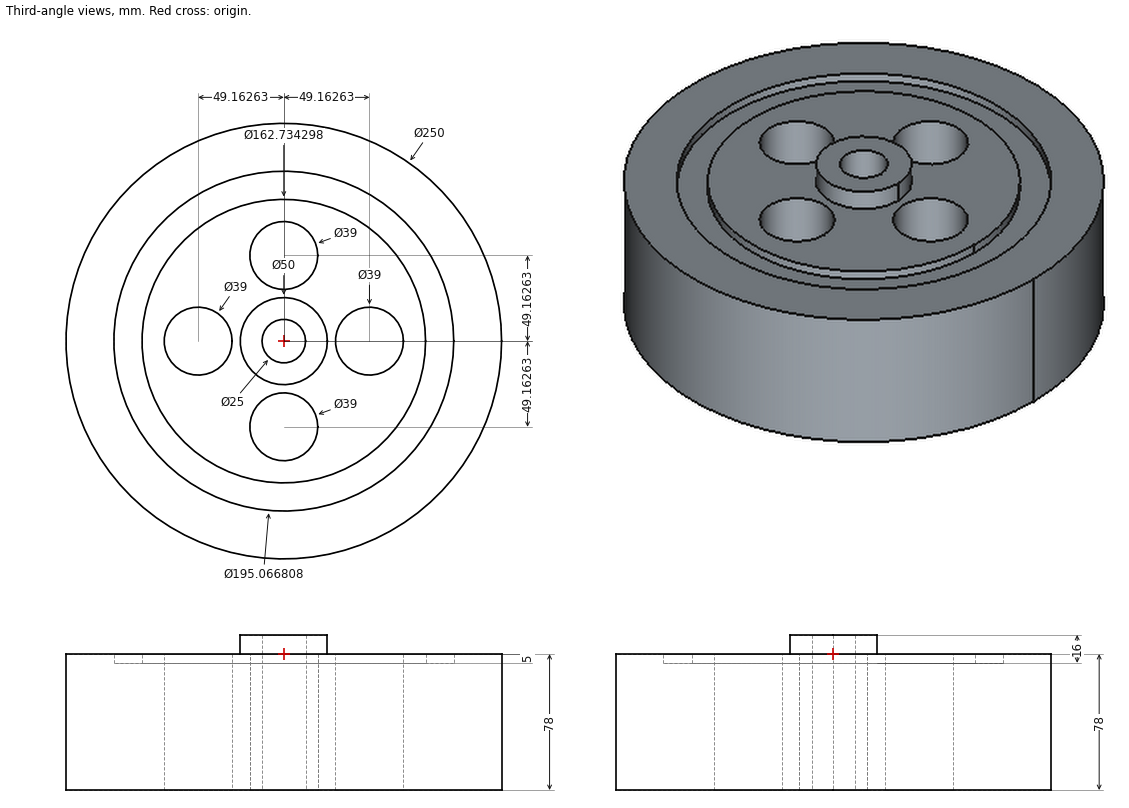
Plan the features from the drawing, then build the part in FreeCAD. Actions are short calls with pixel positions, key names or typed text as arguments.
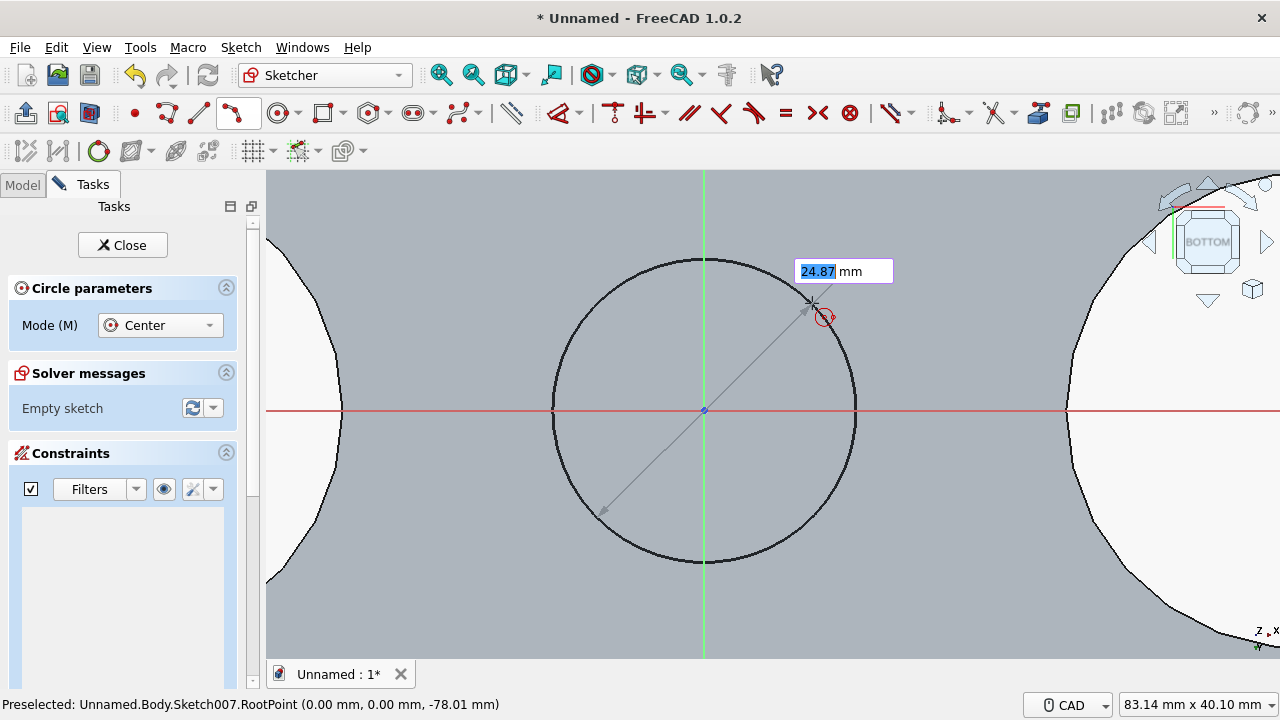
text(25)
key(Return)
key(Escape)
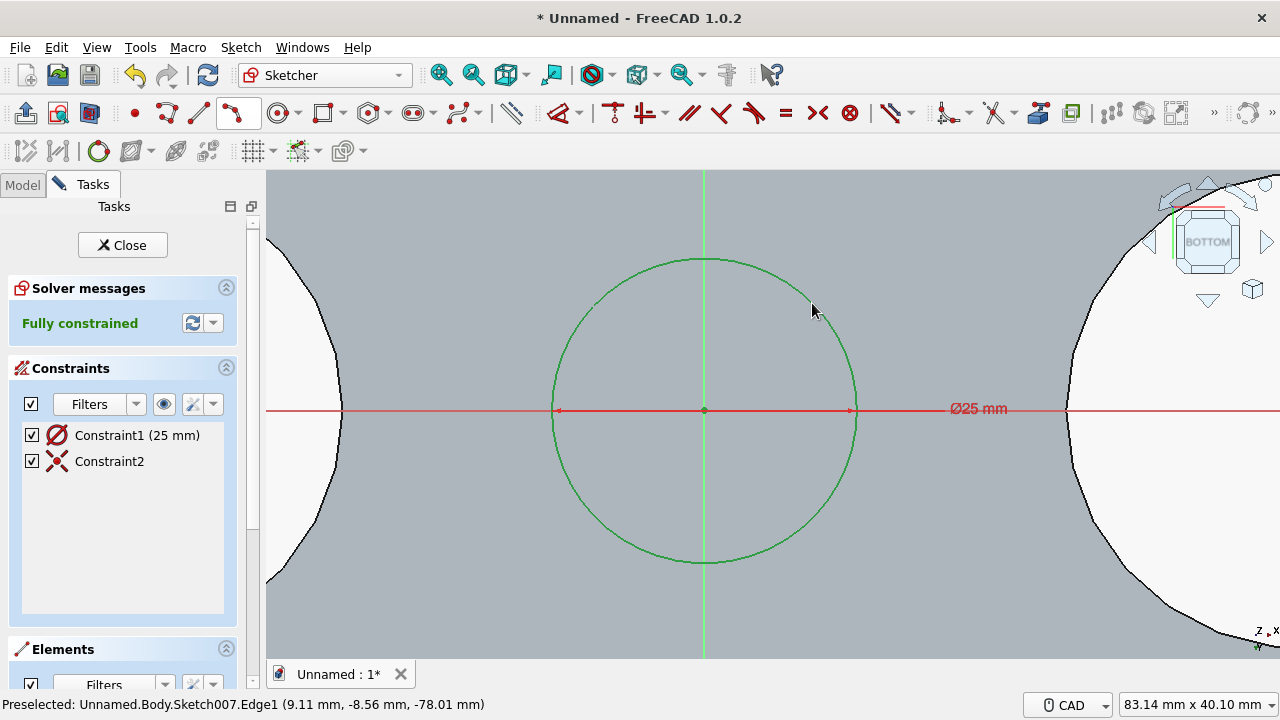
click(123, 245)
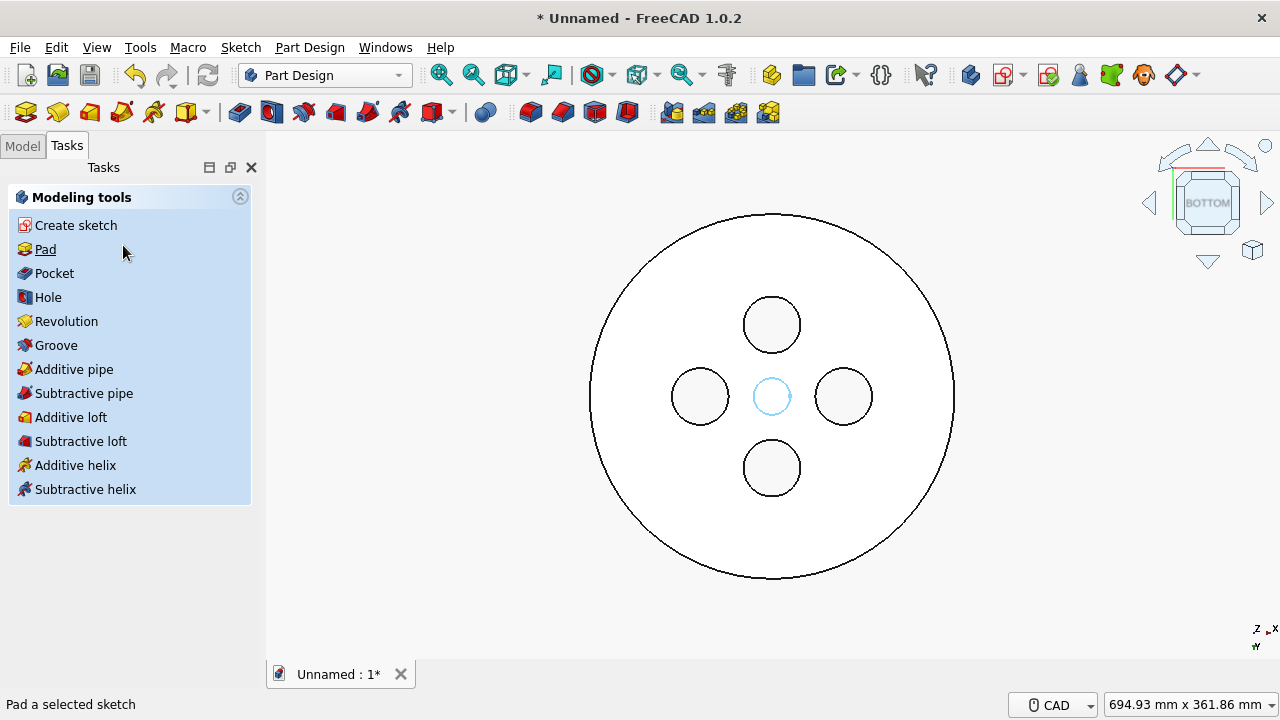
click(240, 112)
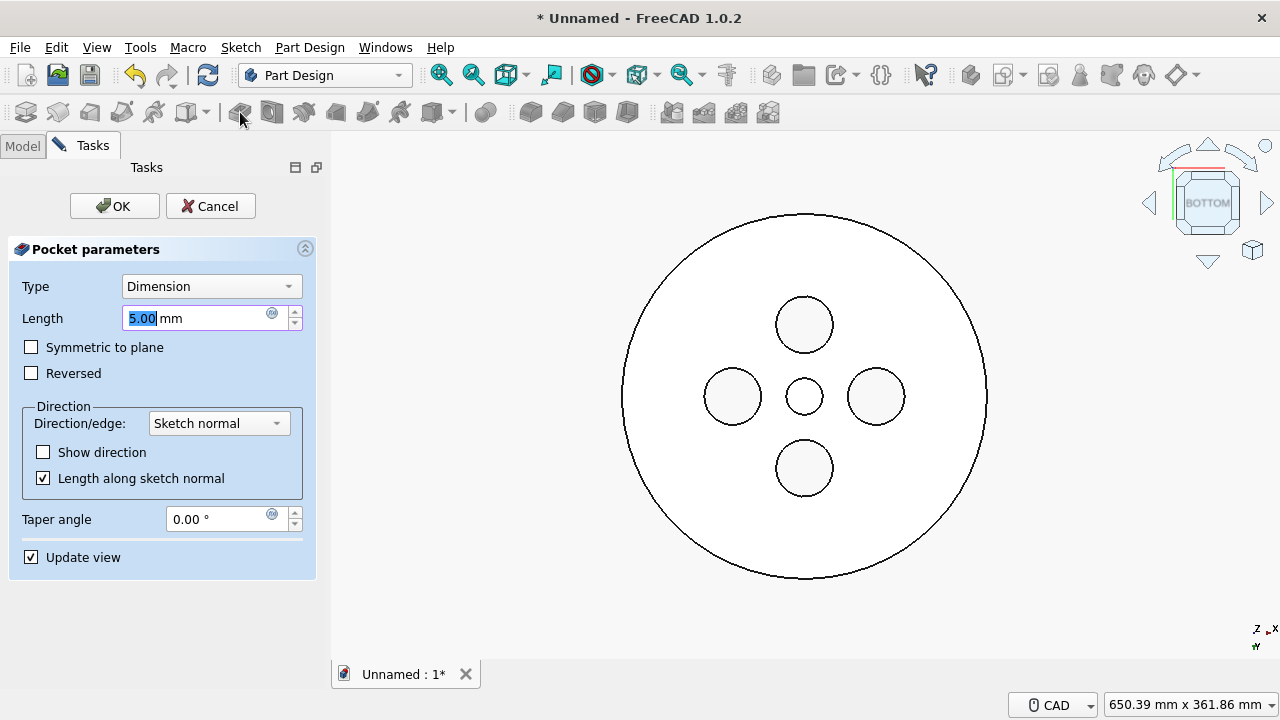
text(78)
key(Tab)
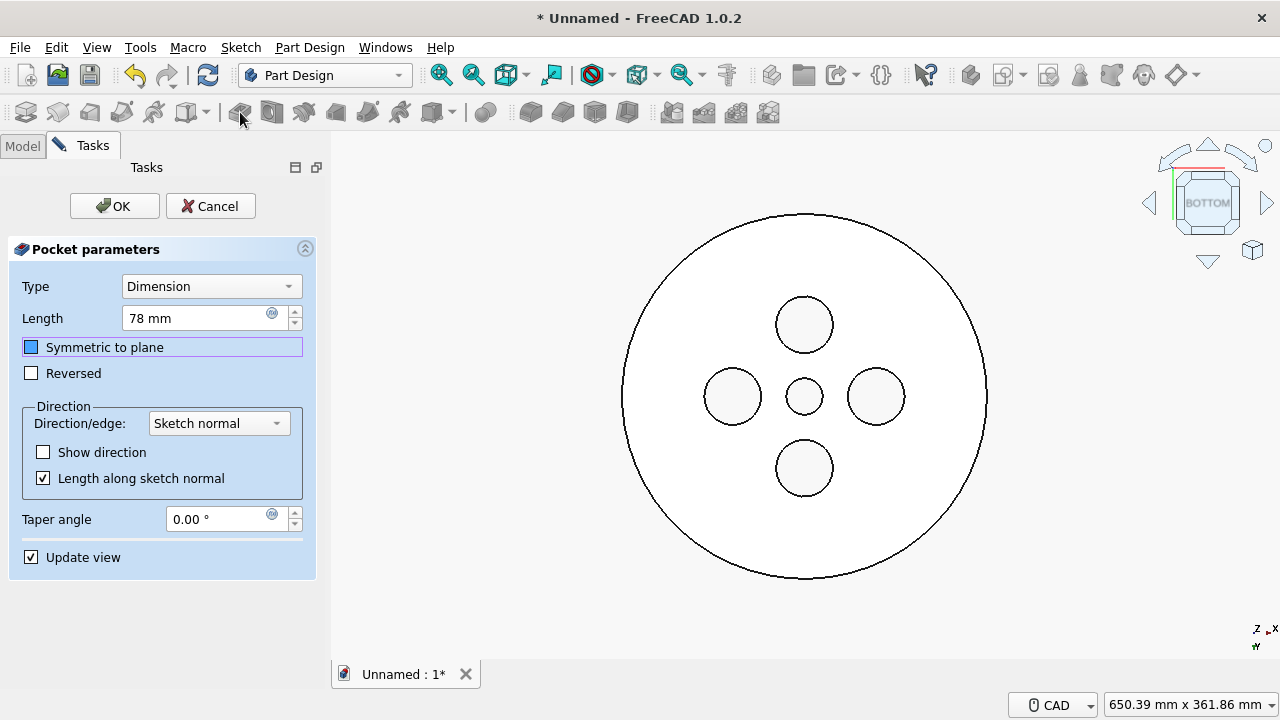
click(115, 206)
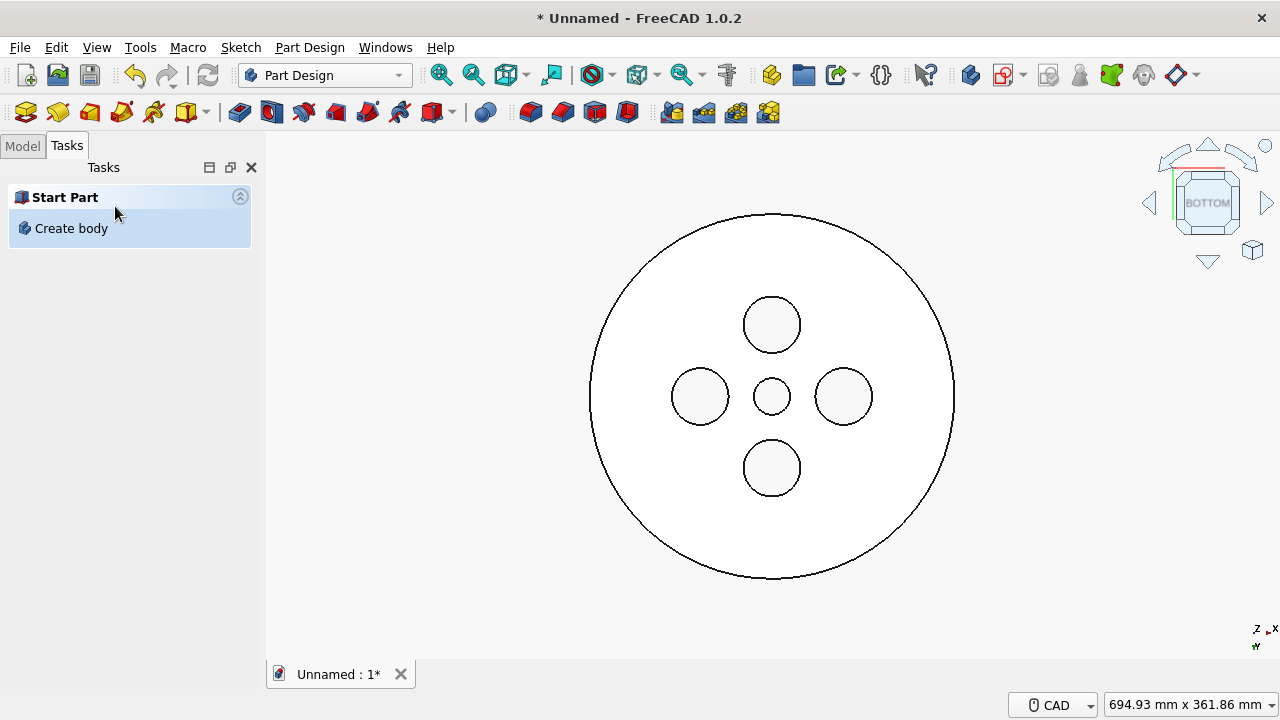
key(0)